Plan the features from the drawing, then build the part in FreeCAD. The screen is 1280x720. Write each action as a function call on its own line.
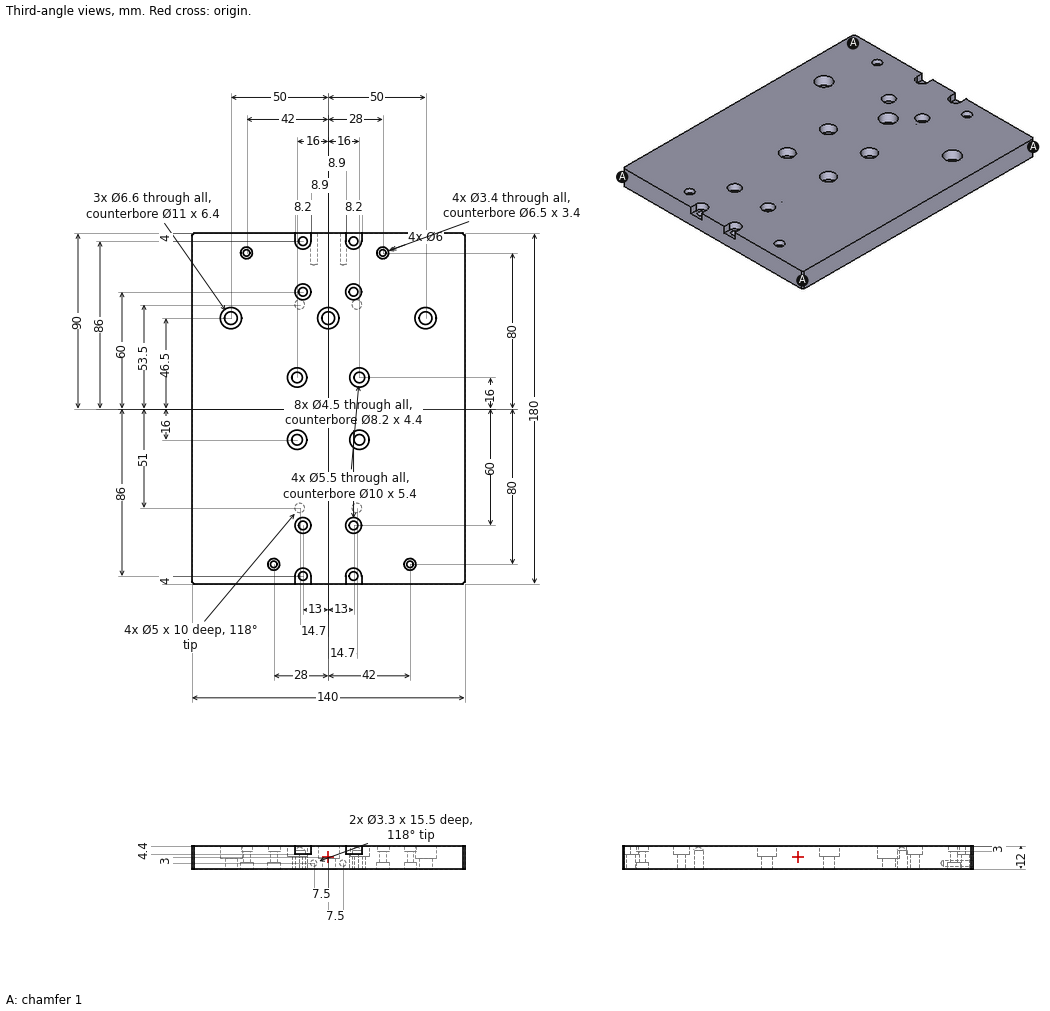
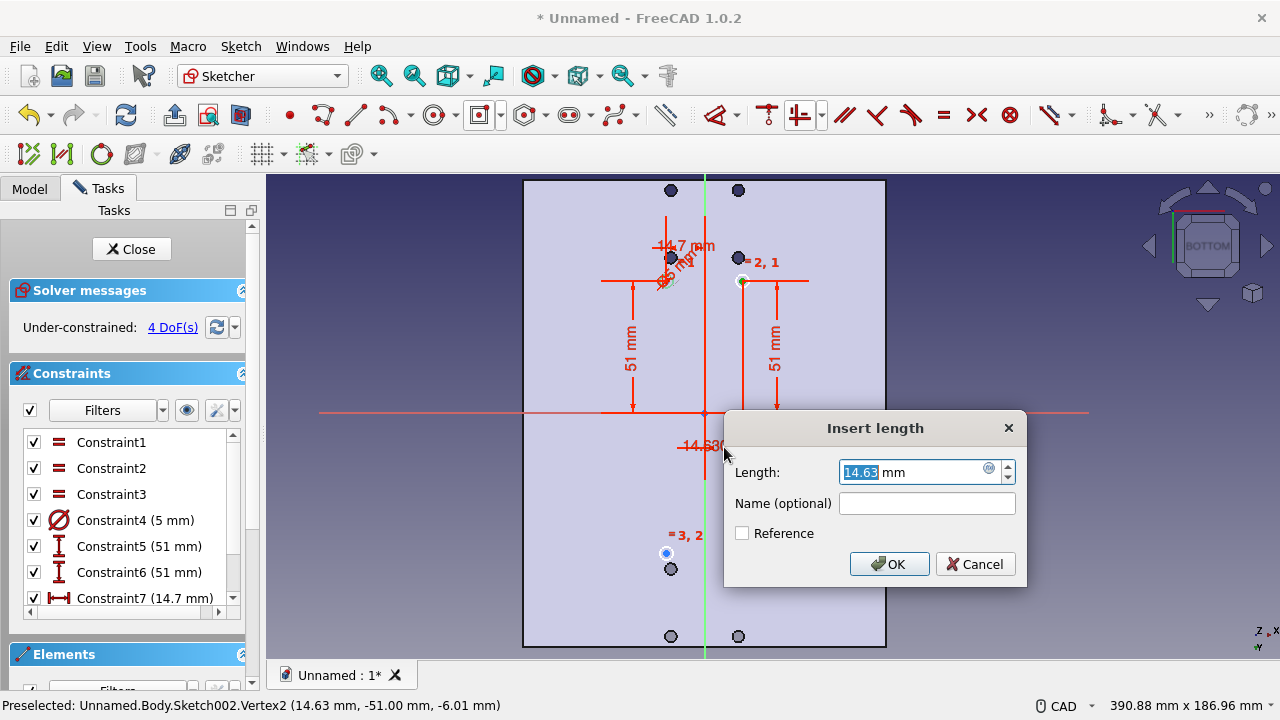
text(14.7)
key(Return)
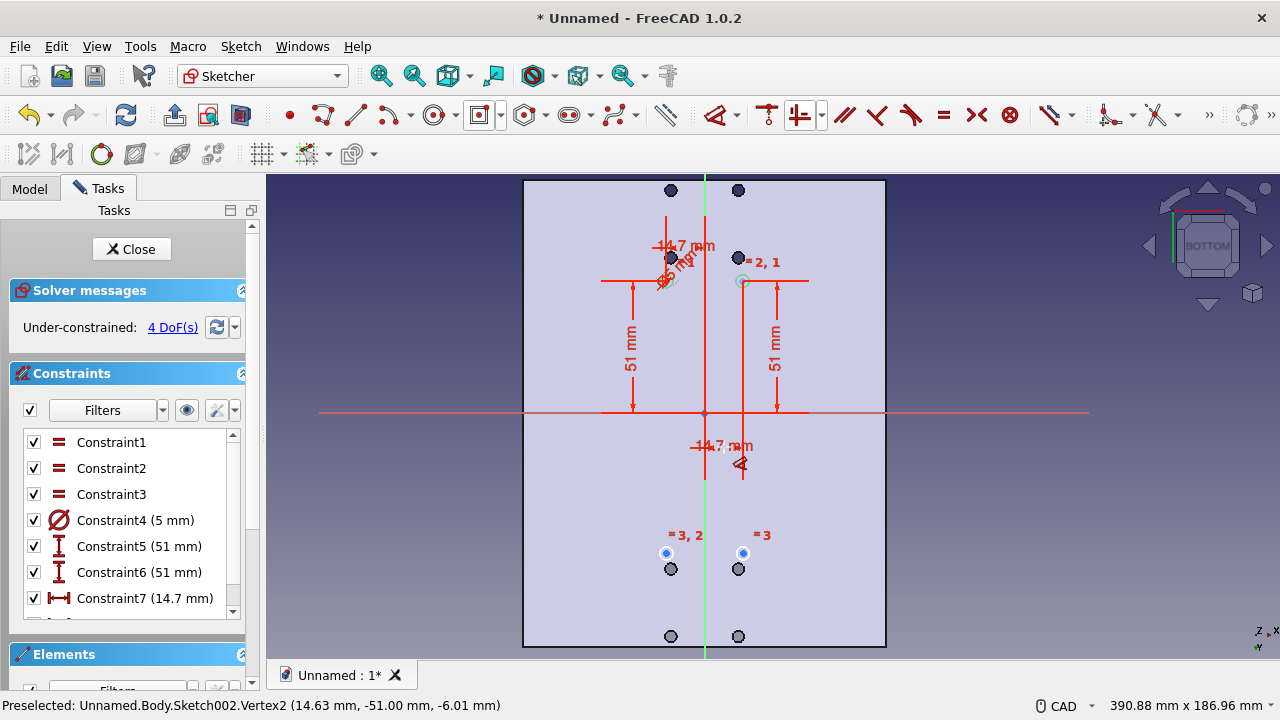
click(667, 553)
click(686, 587)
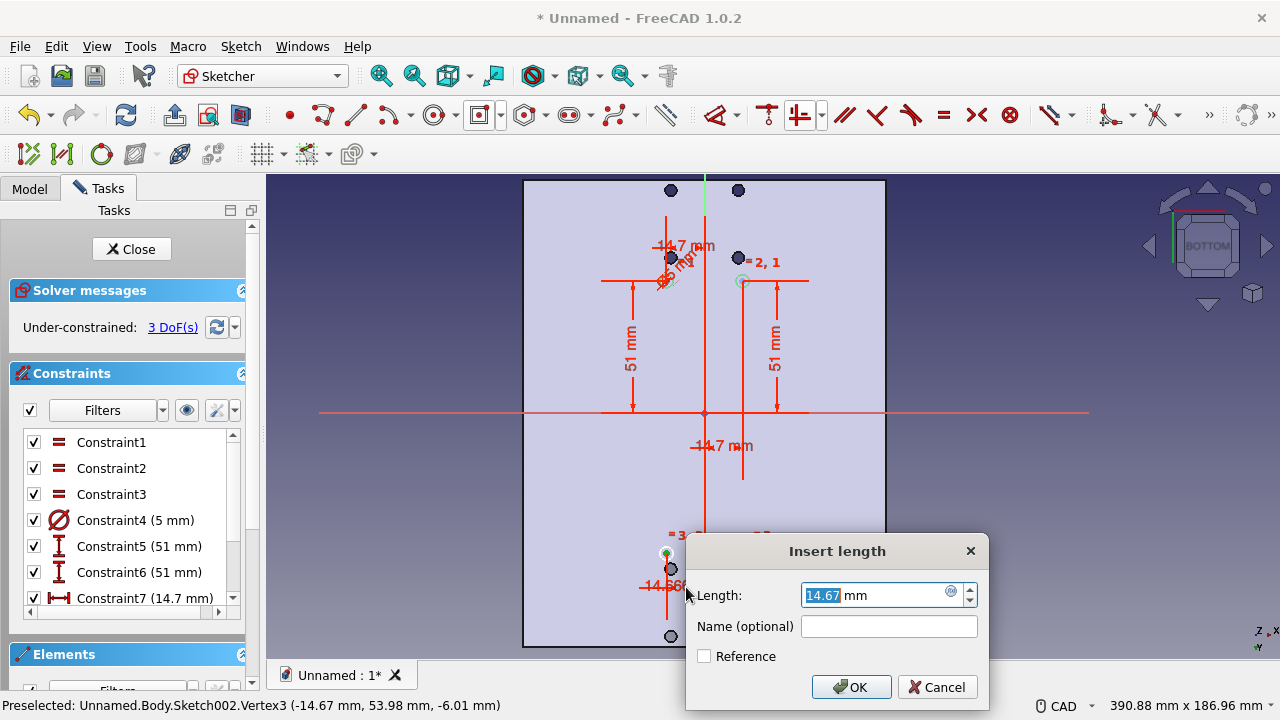
text(14.7)
key(Return)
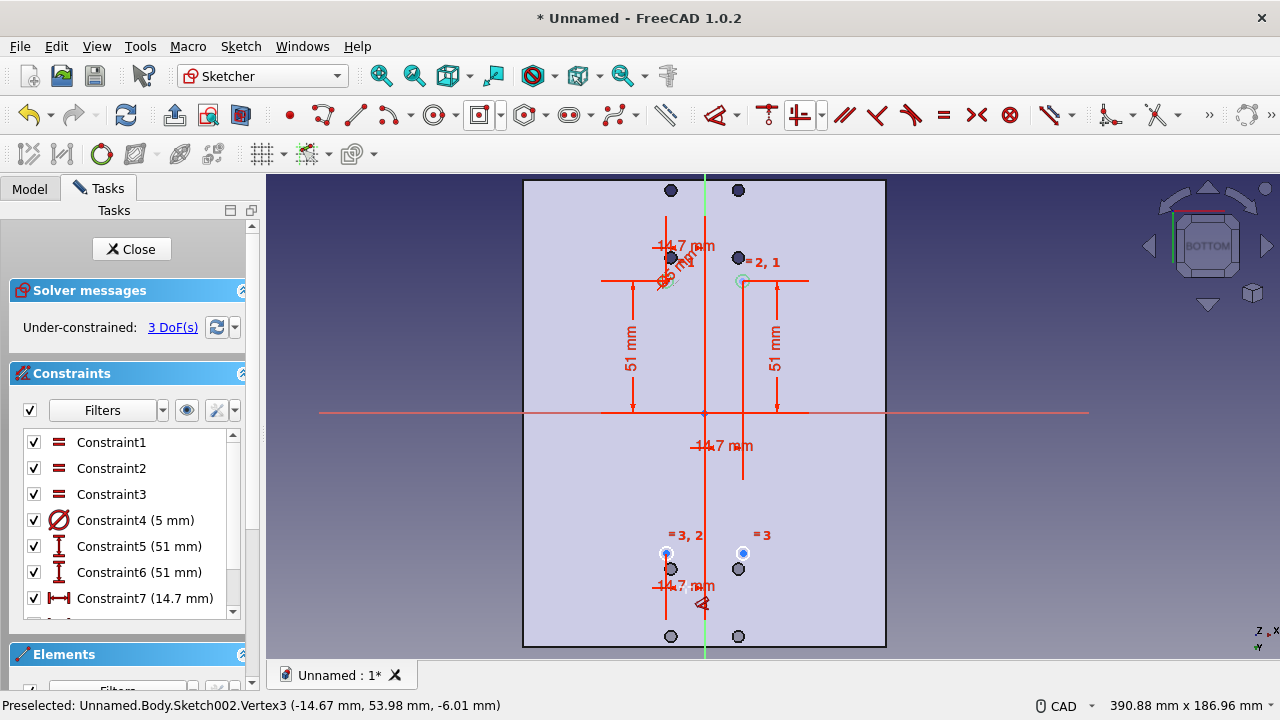
click(666, 553)
click(632, 483)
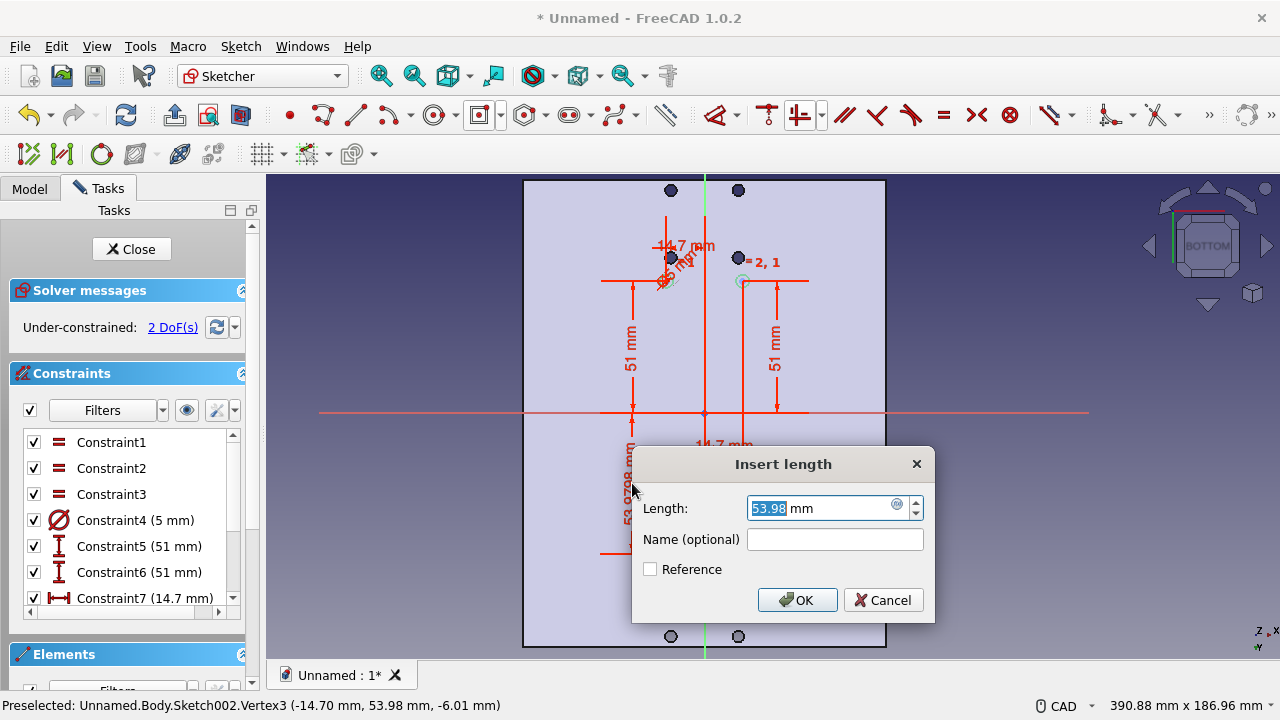
text(53.5)
key(Return)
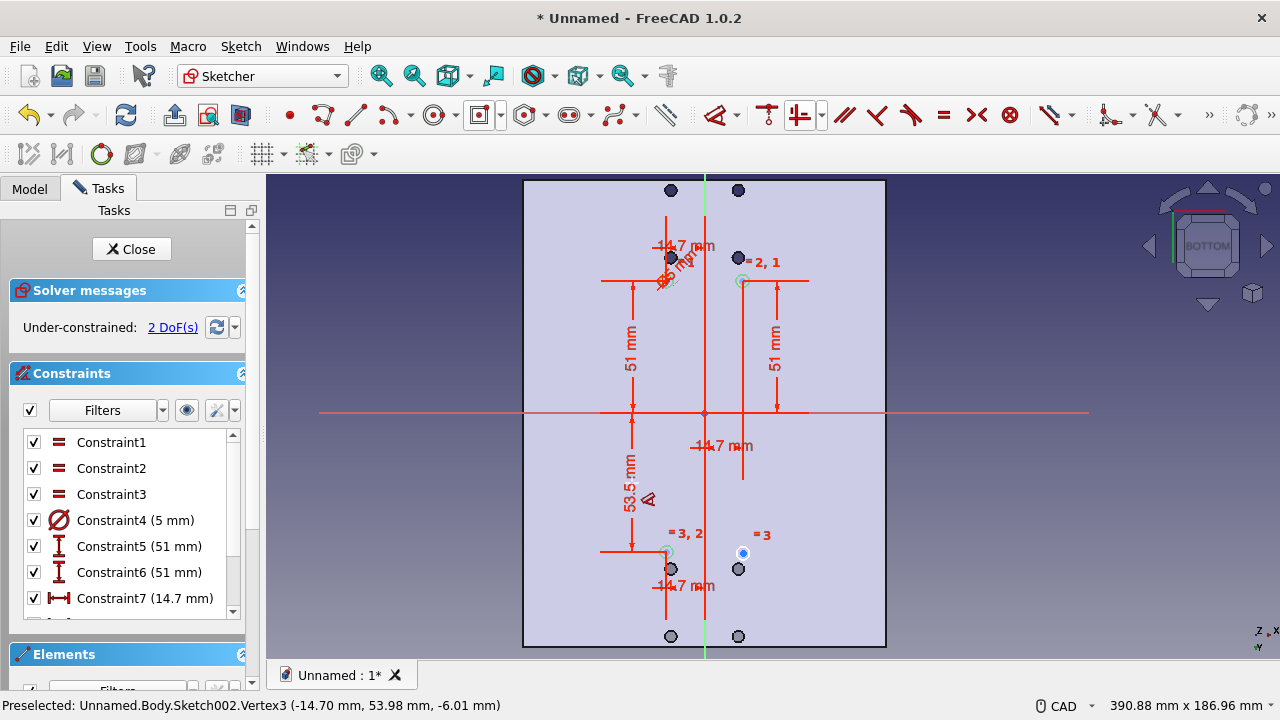
click(743, 553)
click(724, 379)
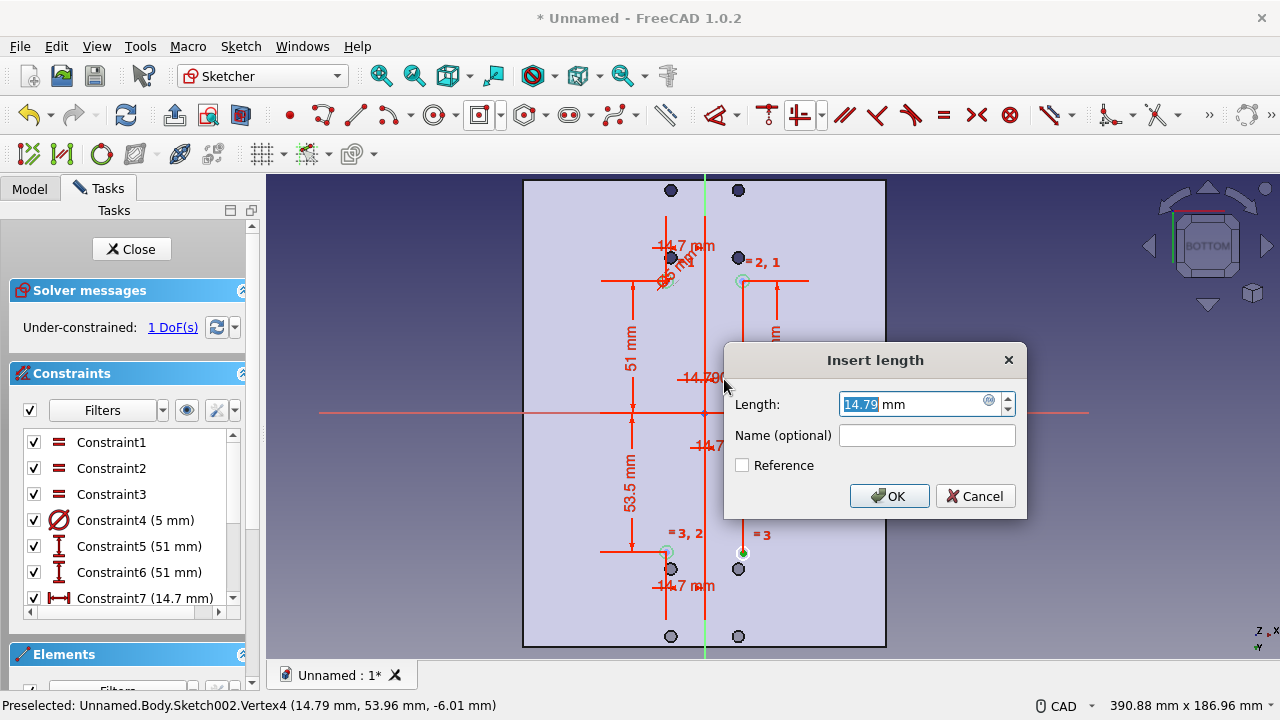
text(14.7)
key(Return)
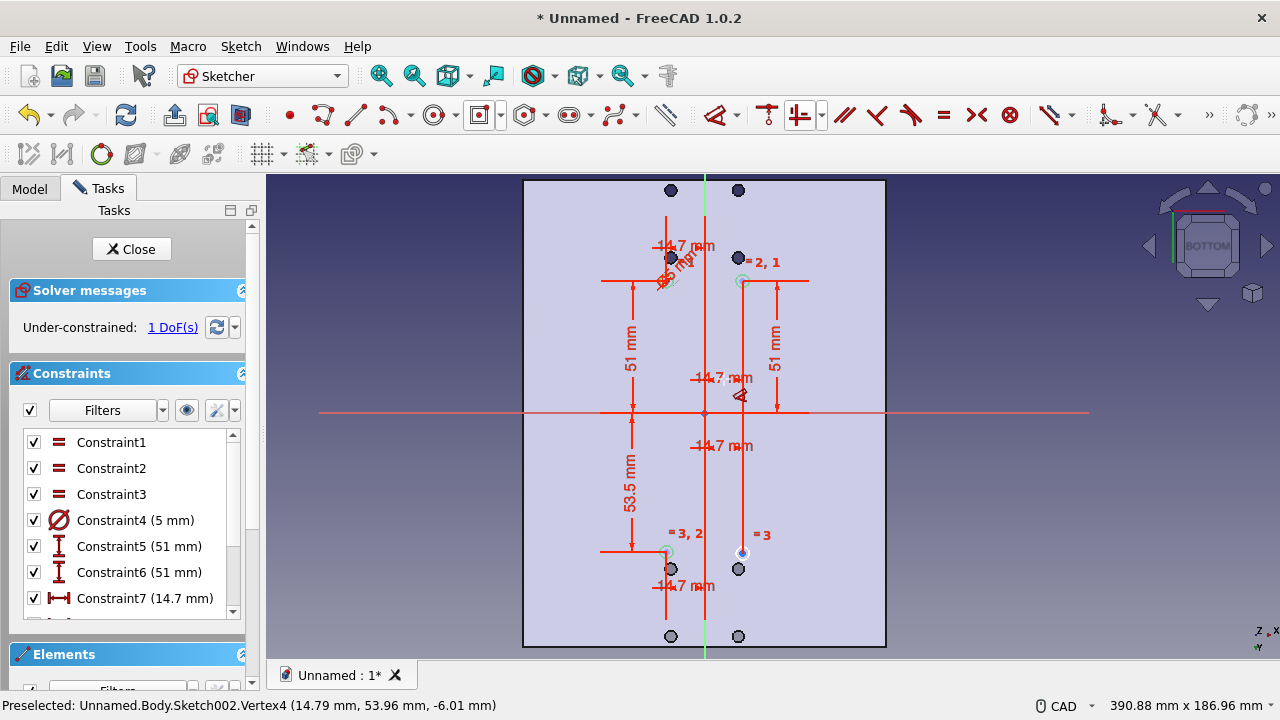
click(743, 553)
click(777, 483)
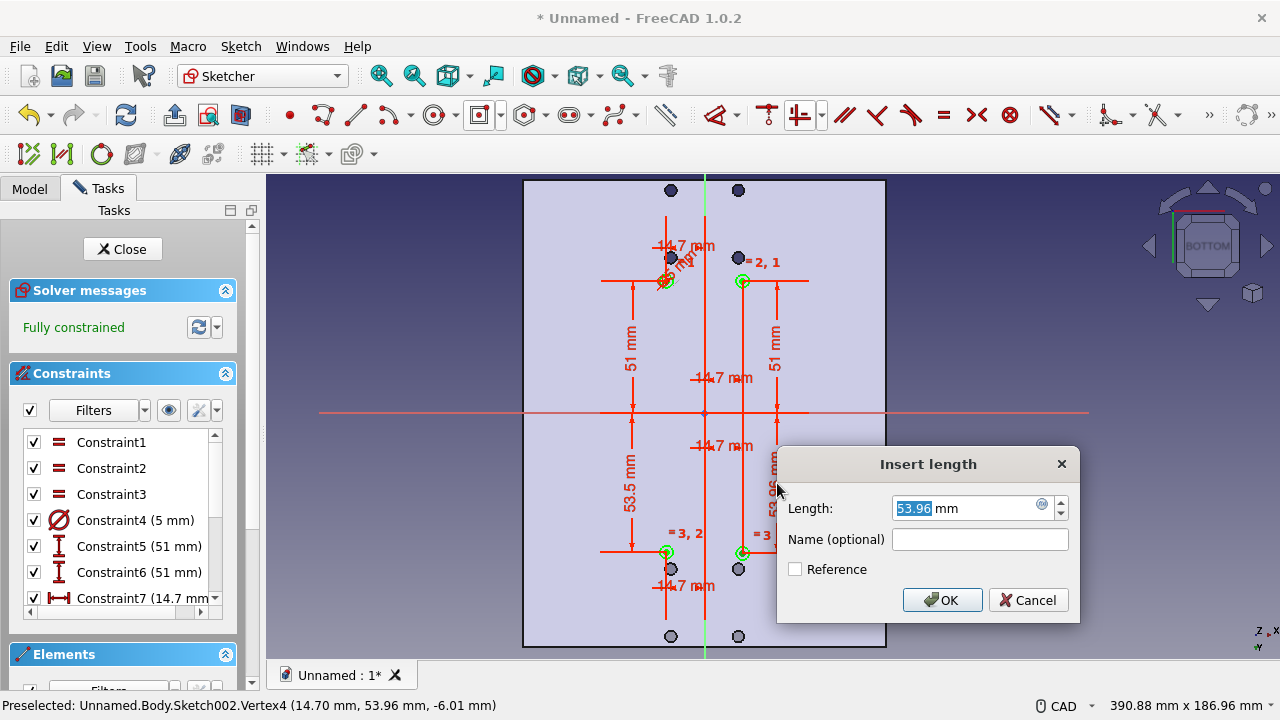
text(53.5)
key(Return)
key(Escape)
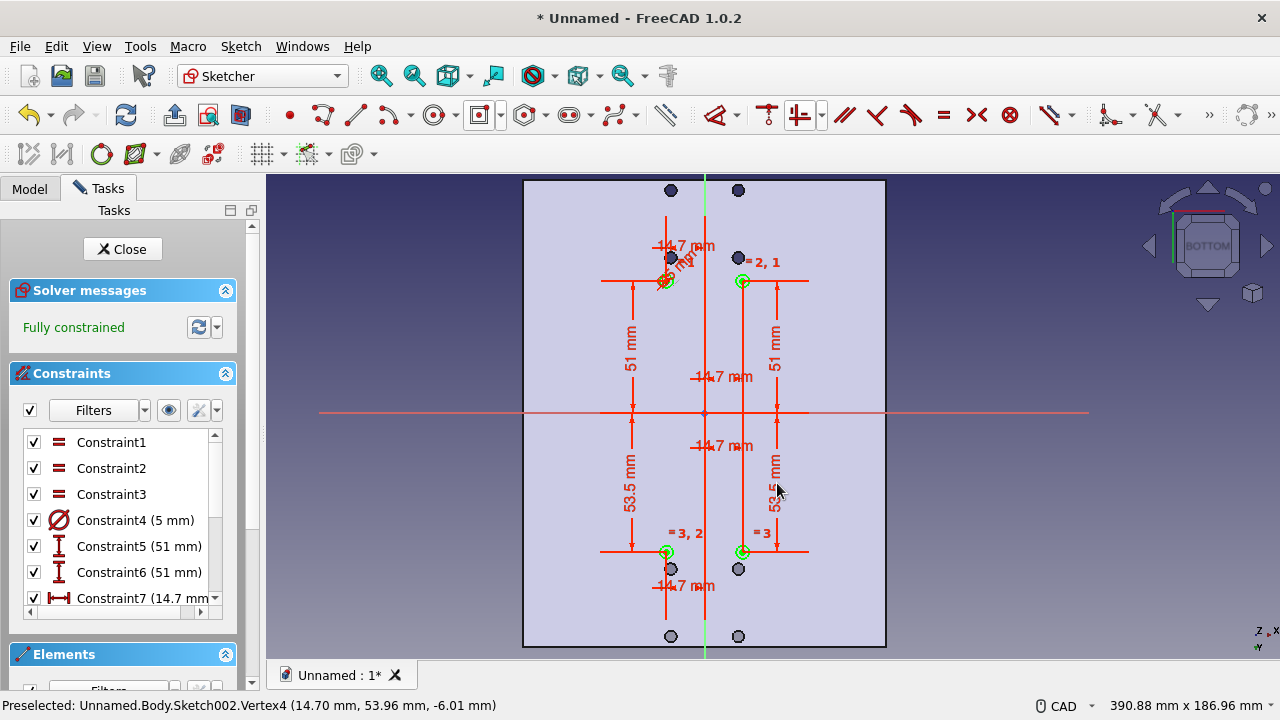
click(123, 249)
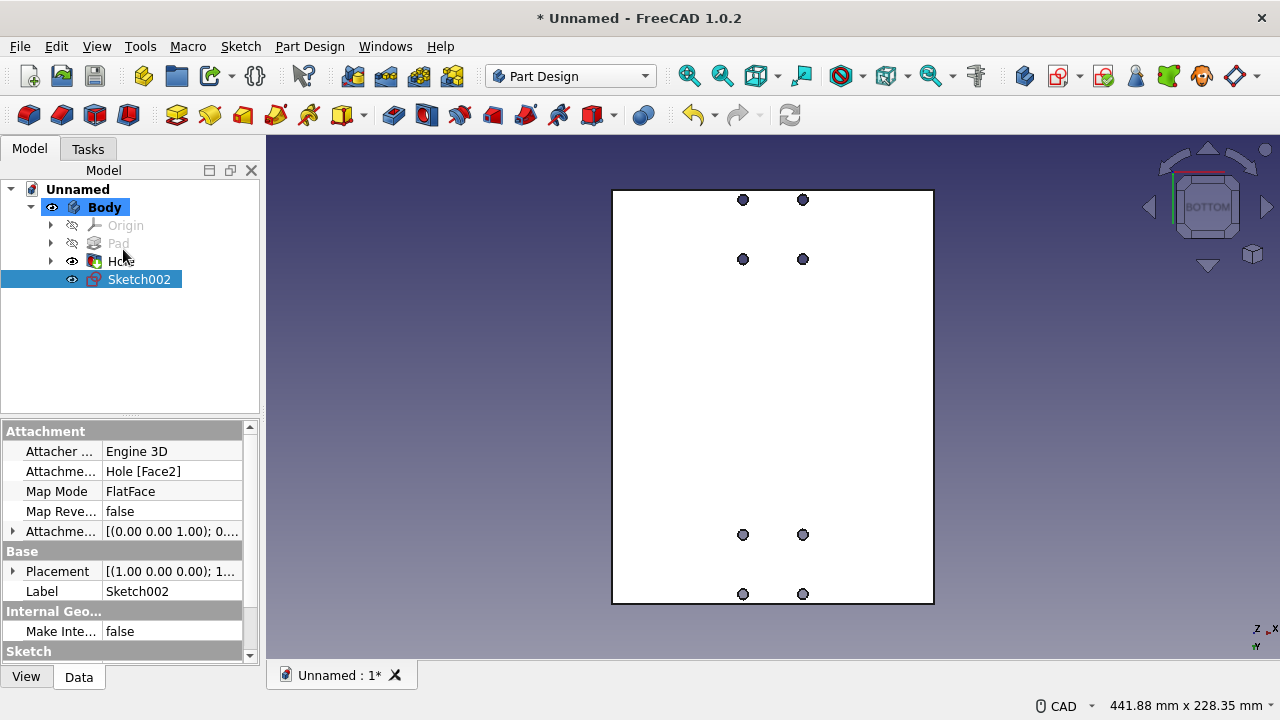
click(427, 116)